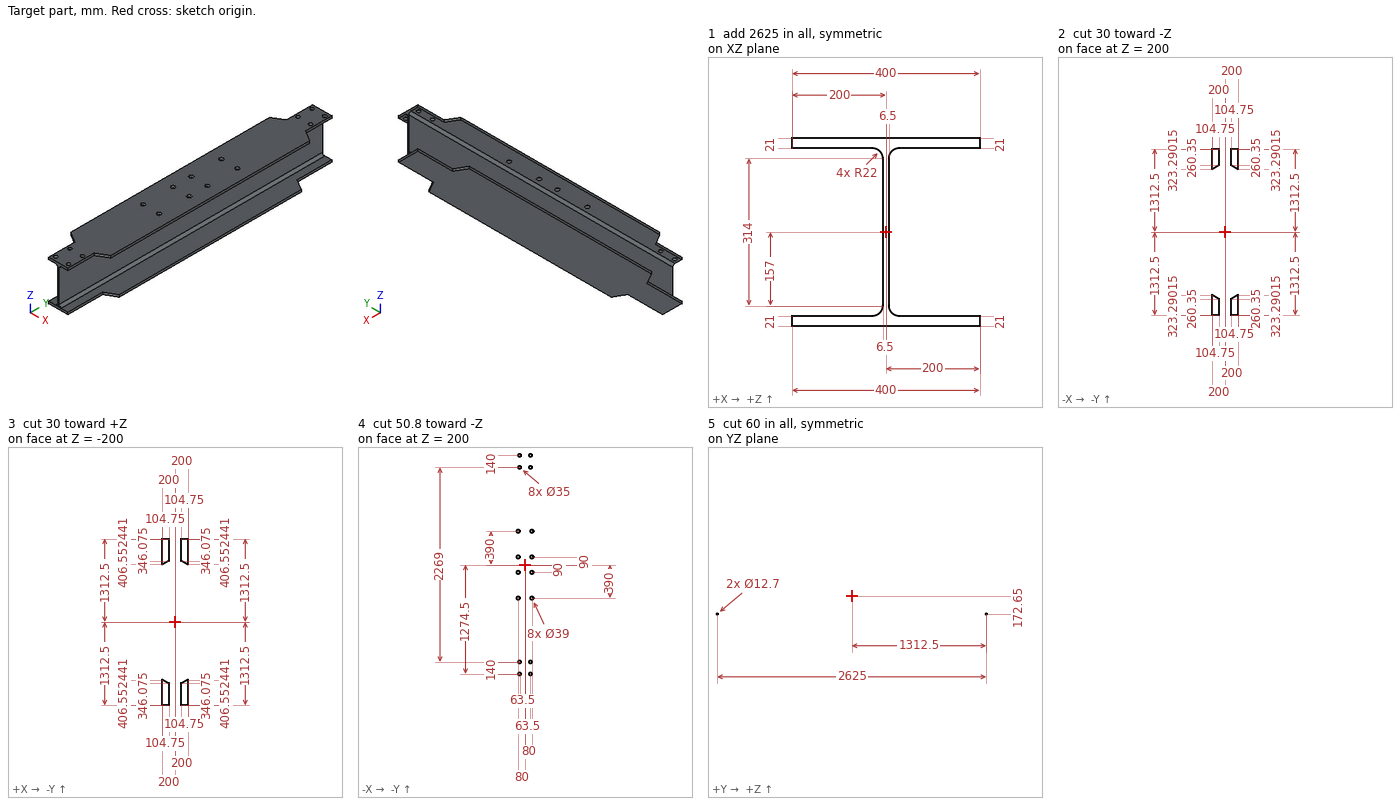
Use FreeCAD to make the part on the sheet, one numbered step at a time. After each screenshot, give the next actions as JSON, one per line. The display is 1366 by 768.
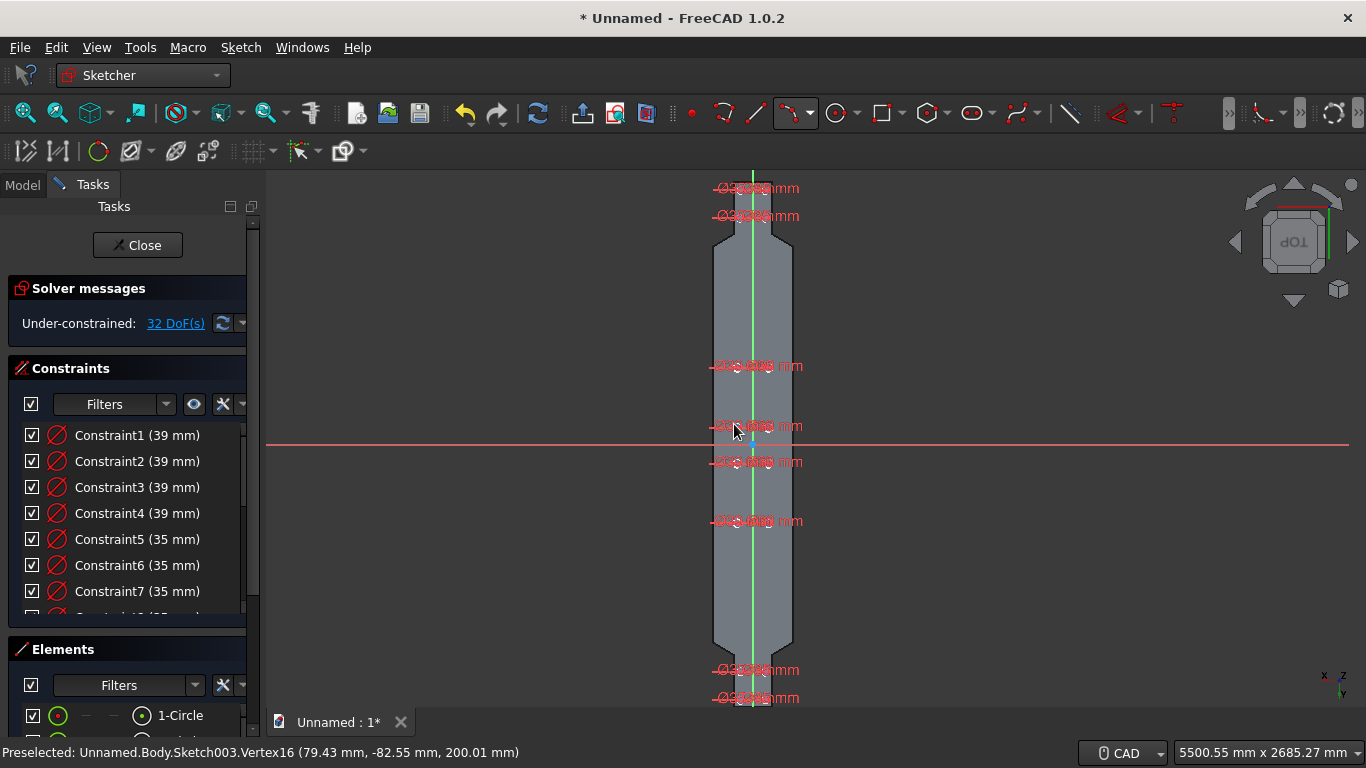
{"action": "left_click", "coordinate": [769, 523]}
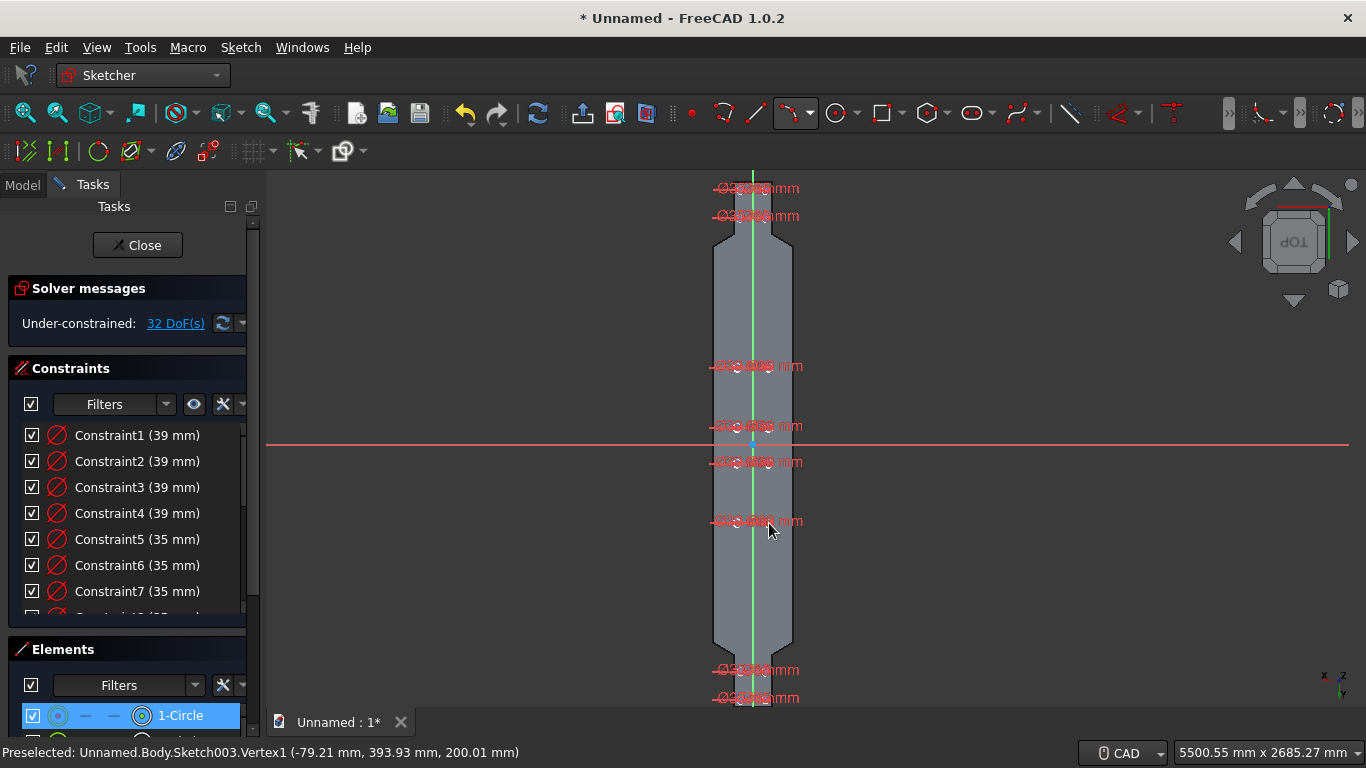
{"action": "left_click", "coordinate": [737, 523]}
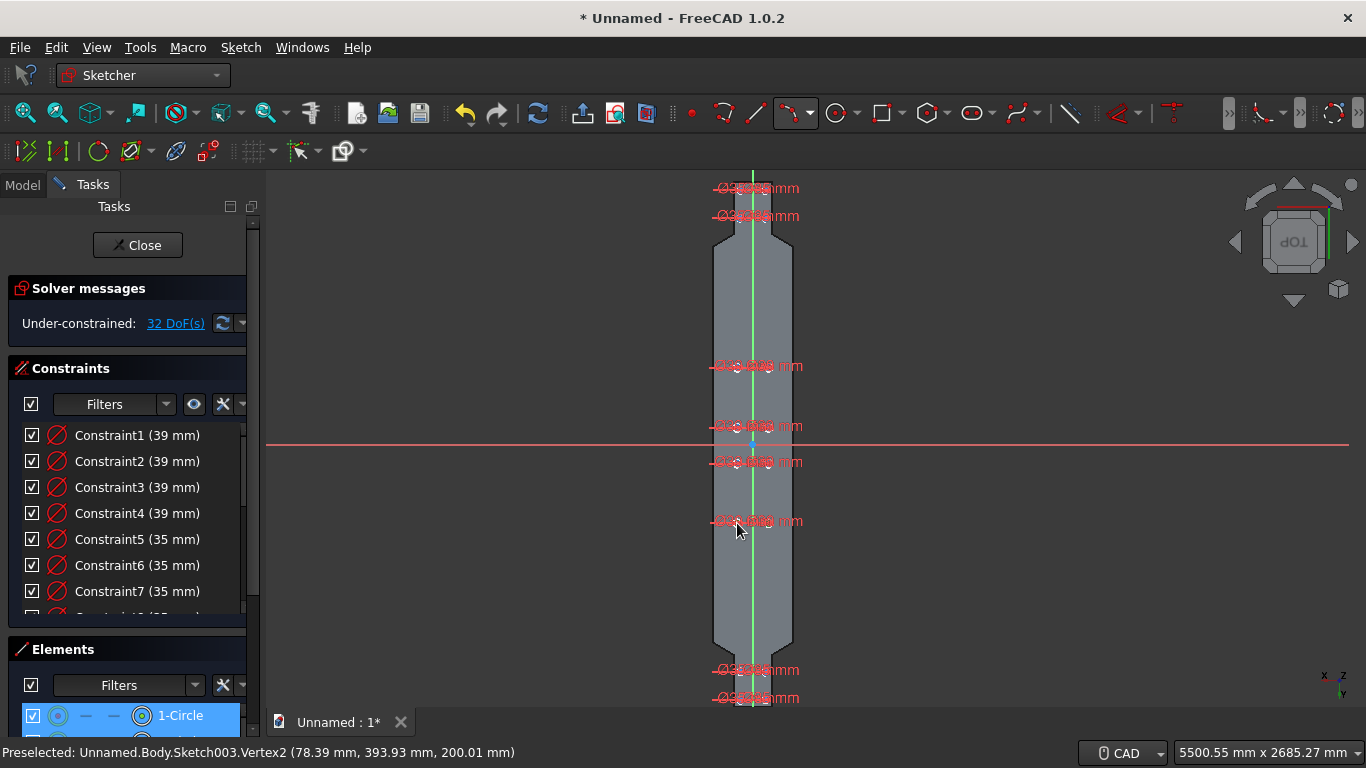
{"action": "key", "text": "h"}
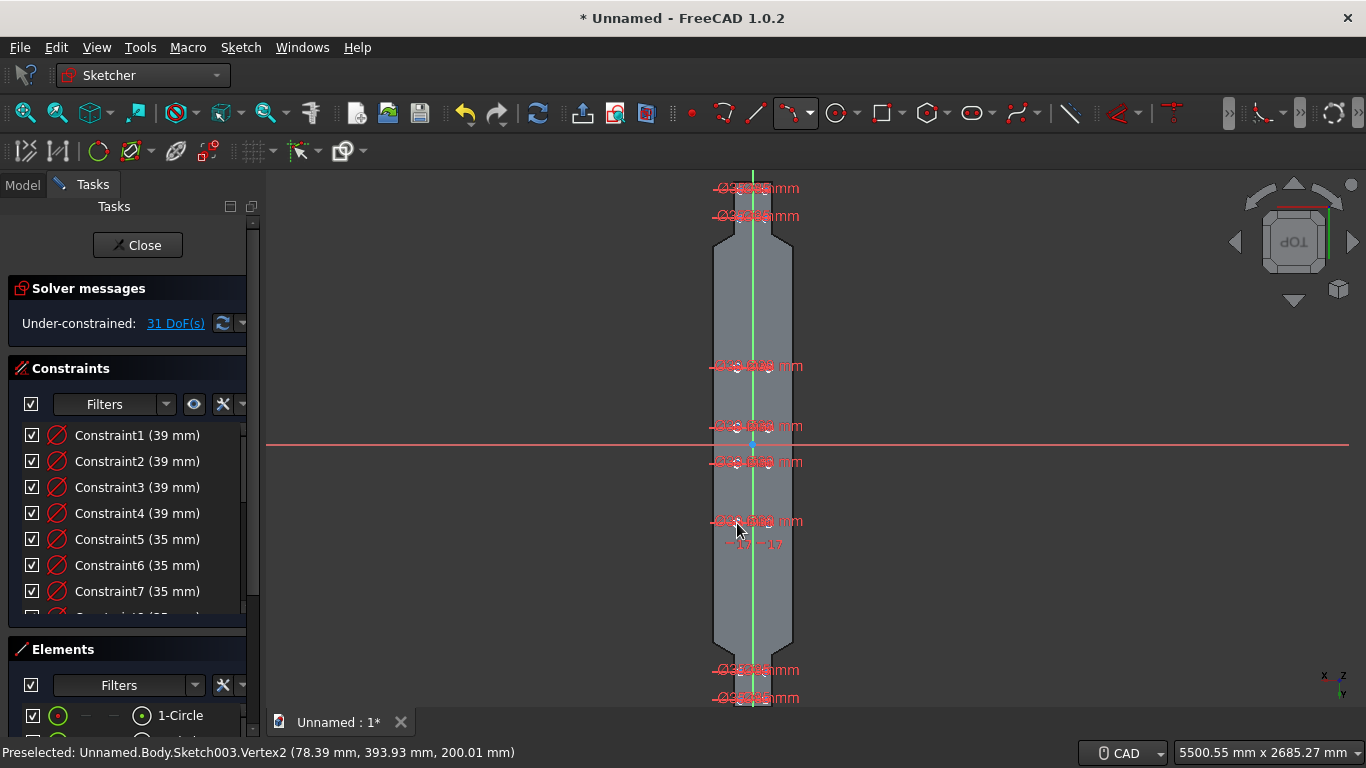
{"action": "left_click", "coordinate": [737, 523]}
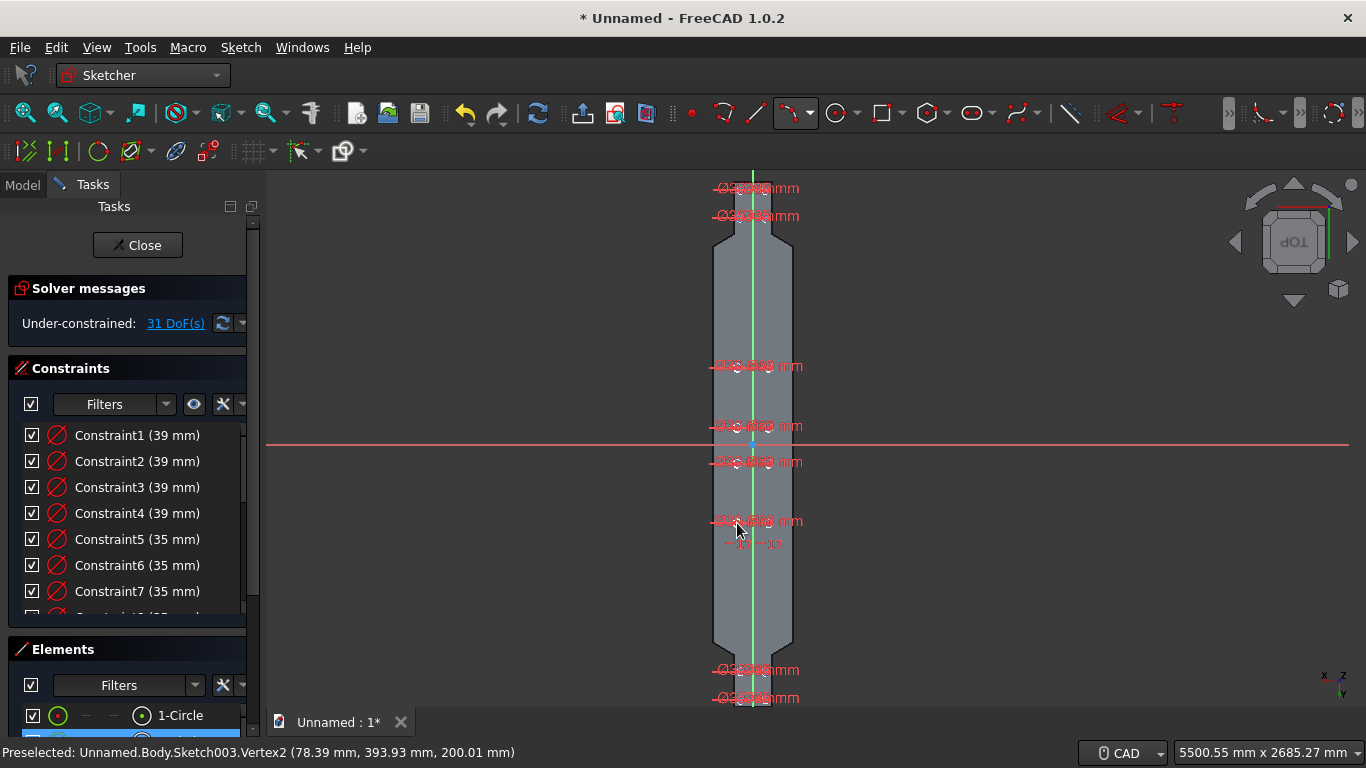
{"action": "left_click", "coordinate": [737, 368]}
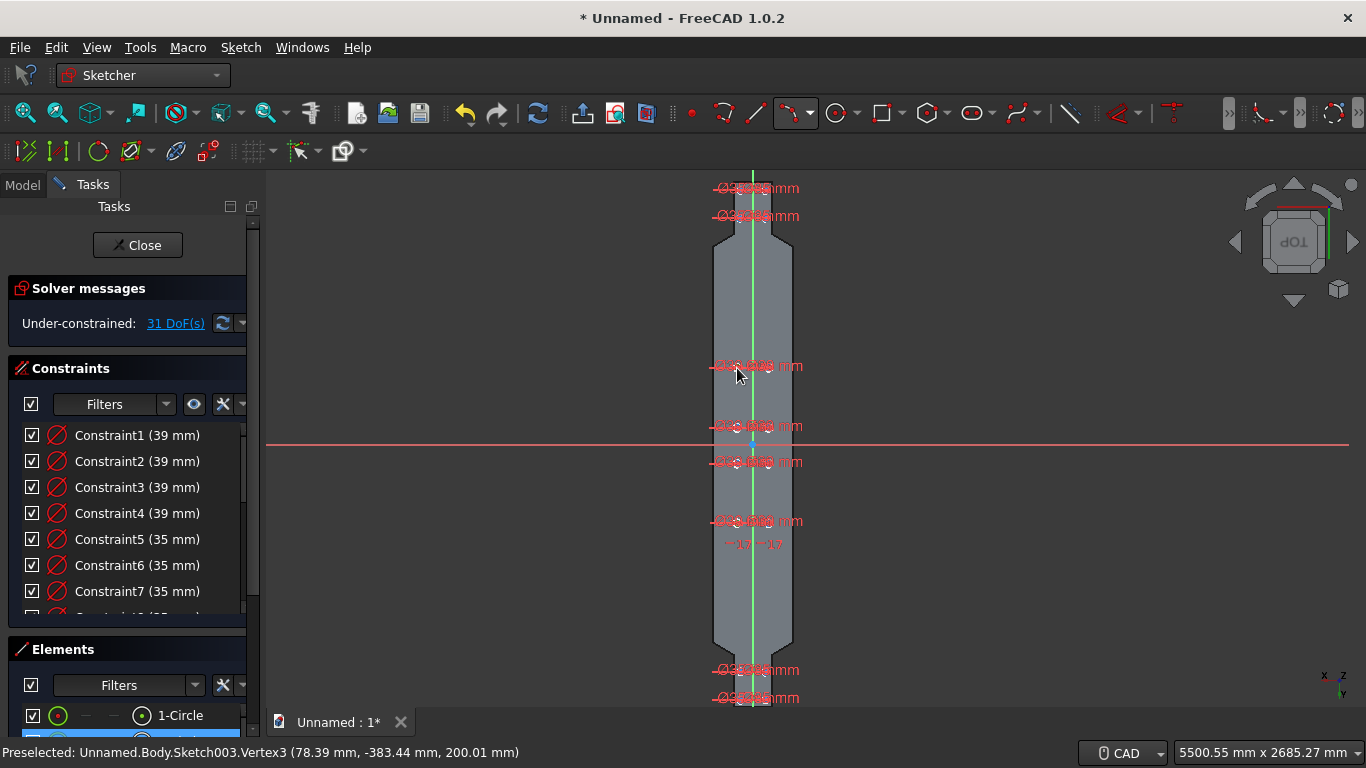
{"action": "key", "text": "v"}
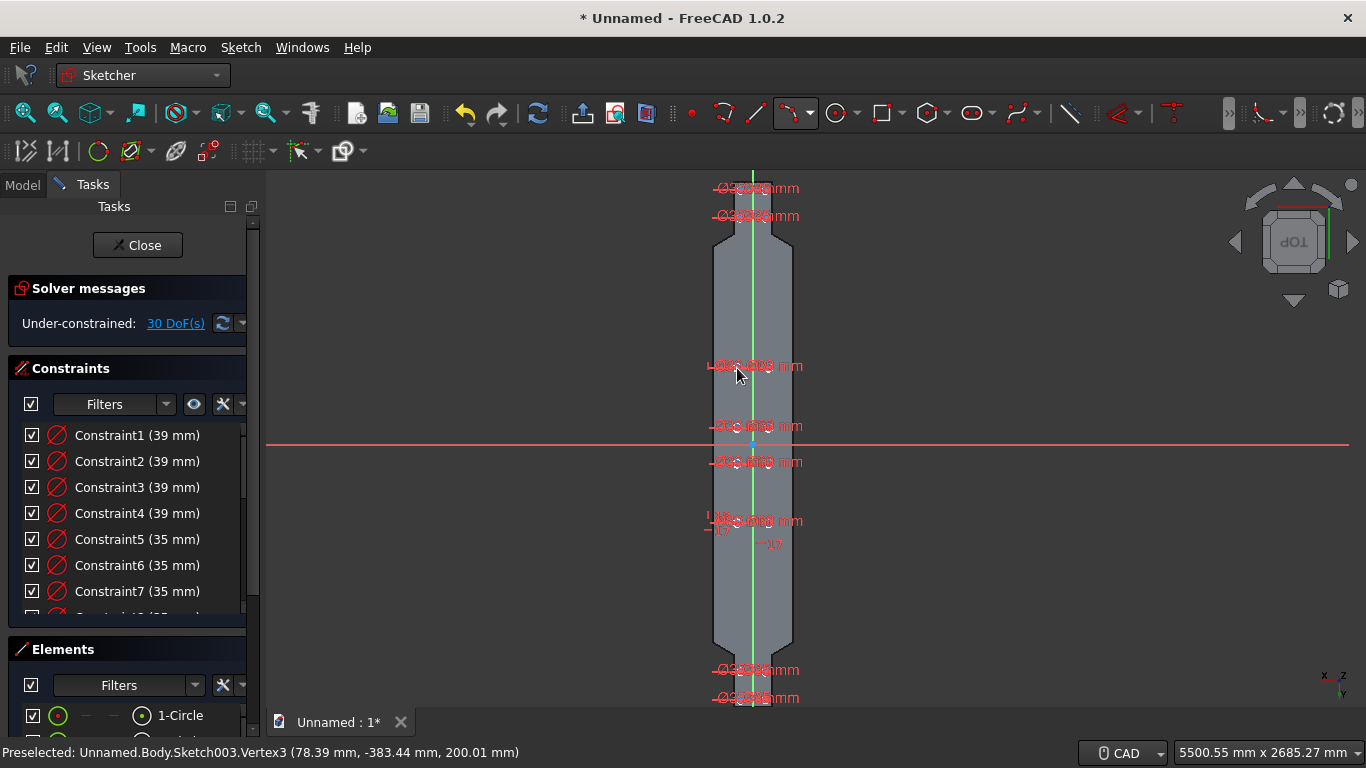
{"action": "left_click", "coordinate": [769, 523]}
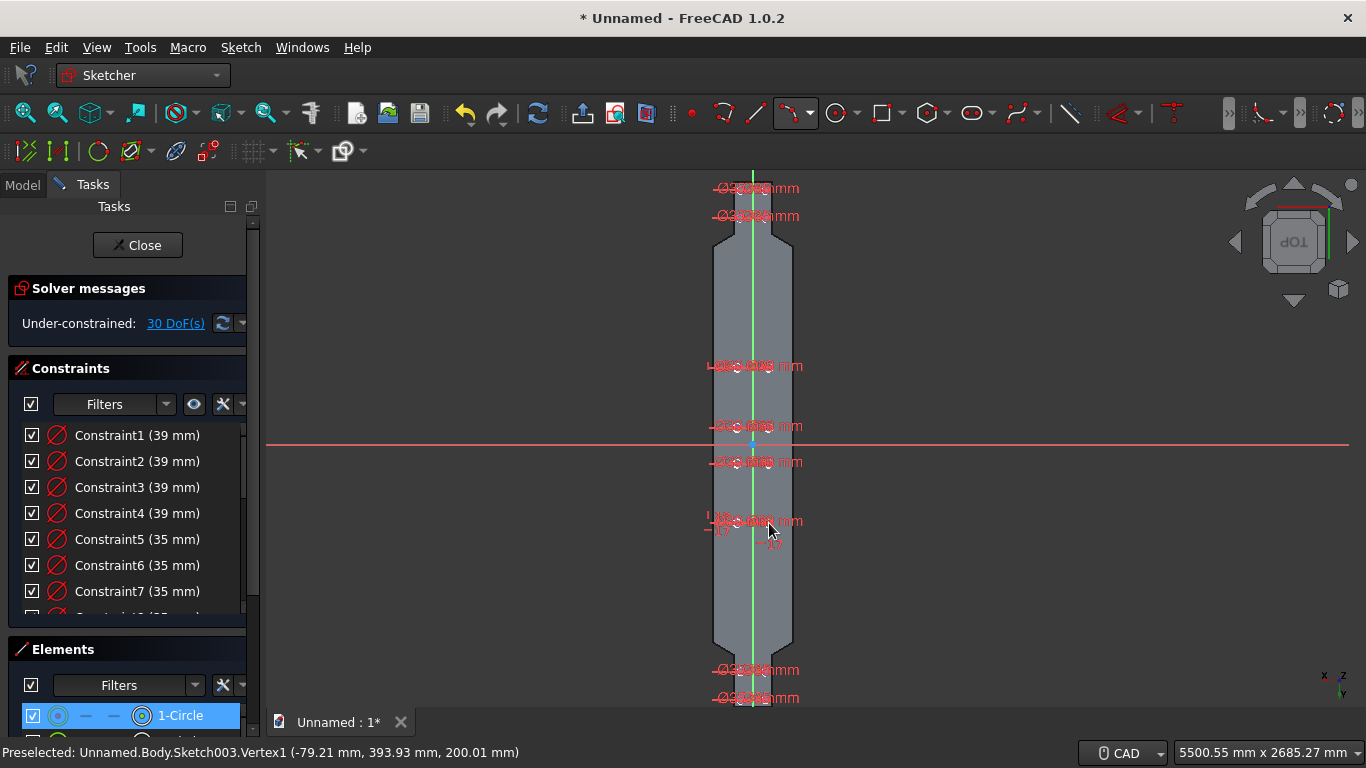
{"action": "left_click", "coordinate": [769, 368]}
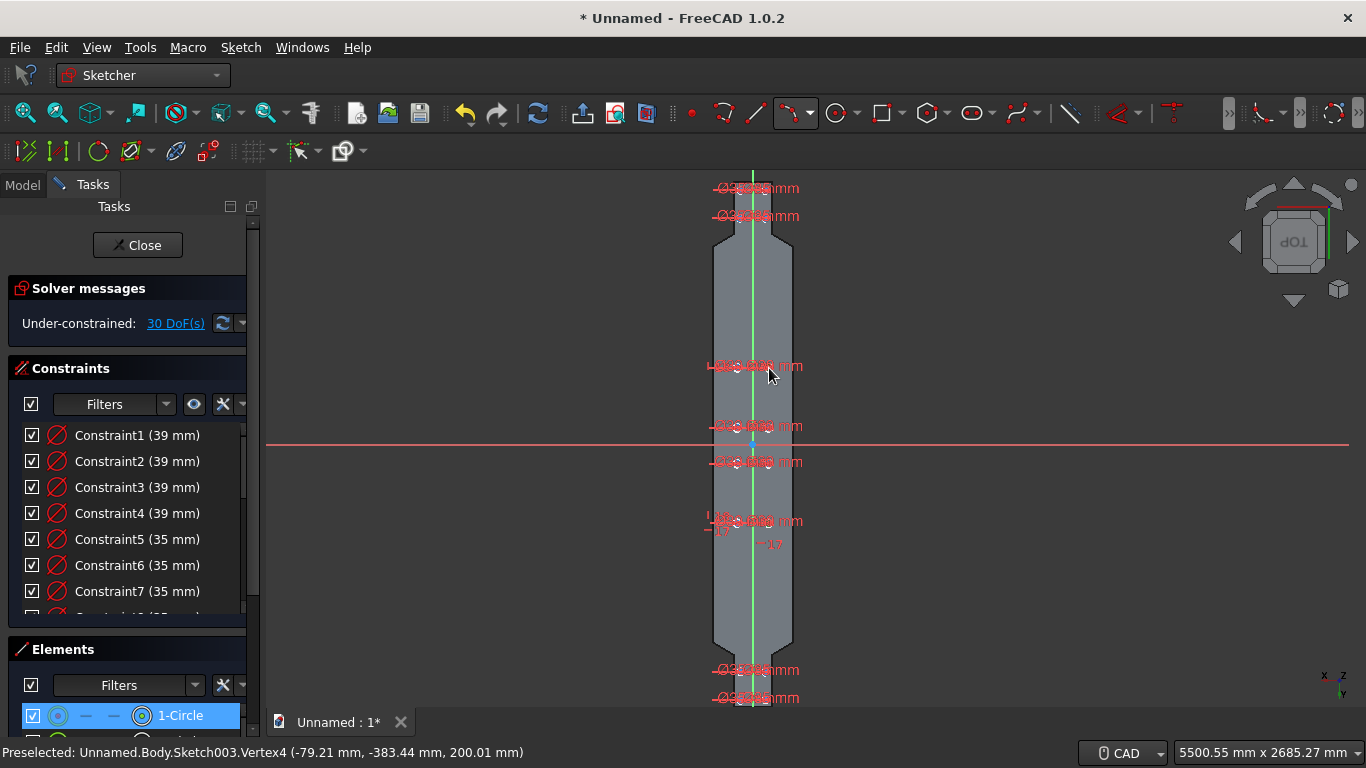
{"action": "key", "text": "v"}